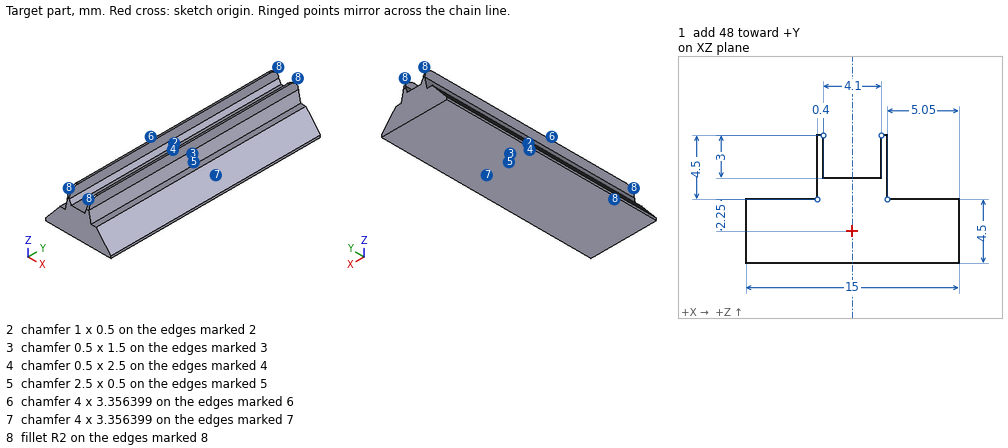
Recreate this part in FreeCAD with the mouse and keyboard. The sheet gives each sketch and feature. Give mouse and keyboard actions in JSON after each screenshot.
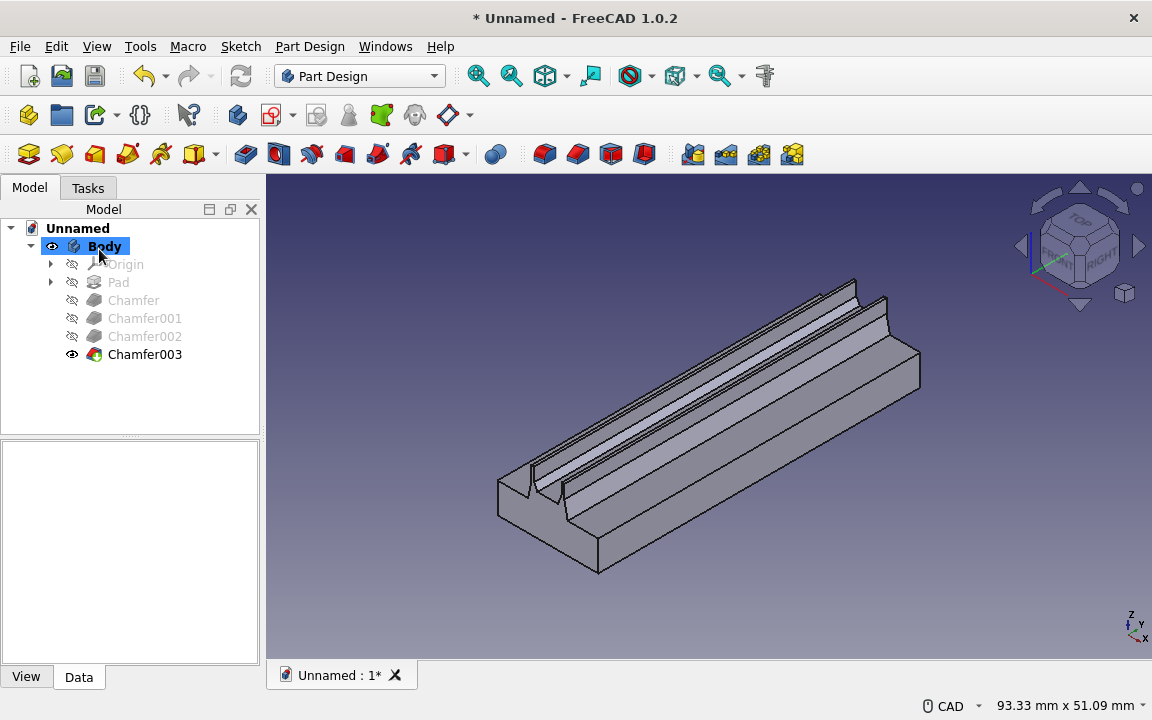
{"action": "key", "text": "2"}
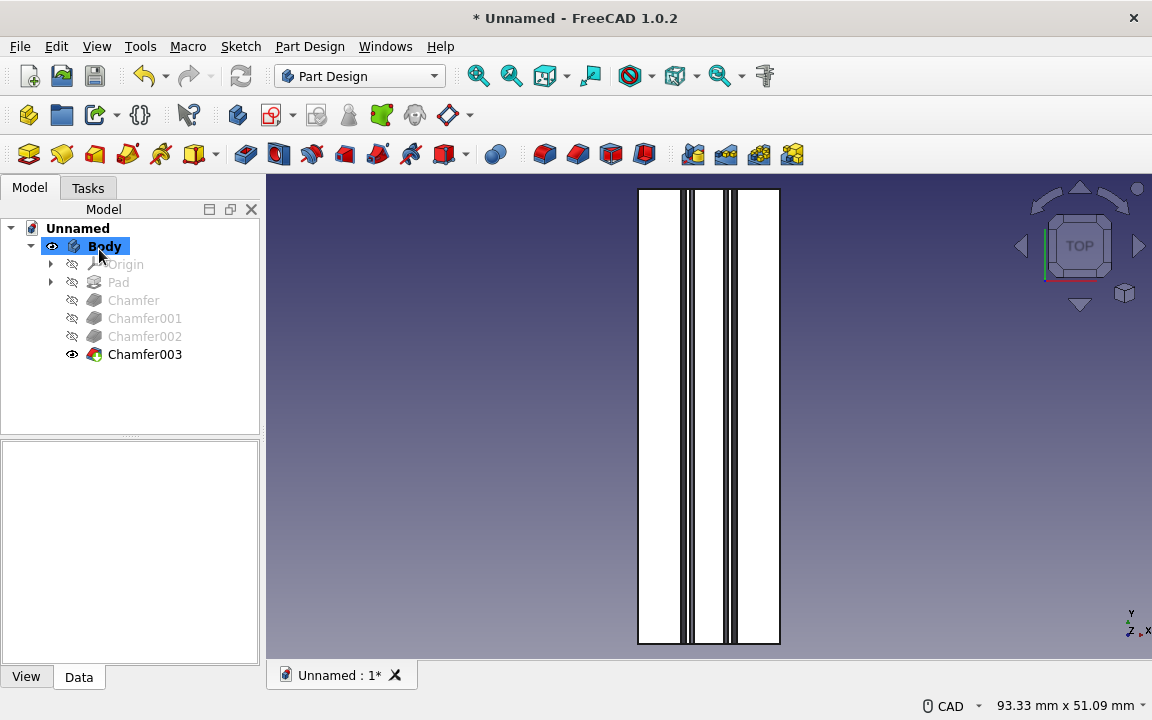
{"action": "left_click", "coordinate": [638, 416]}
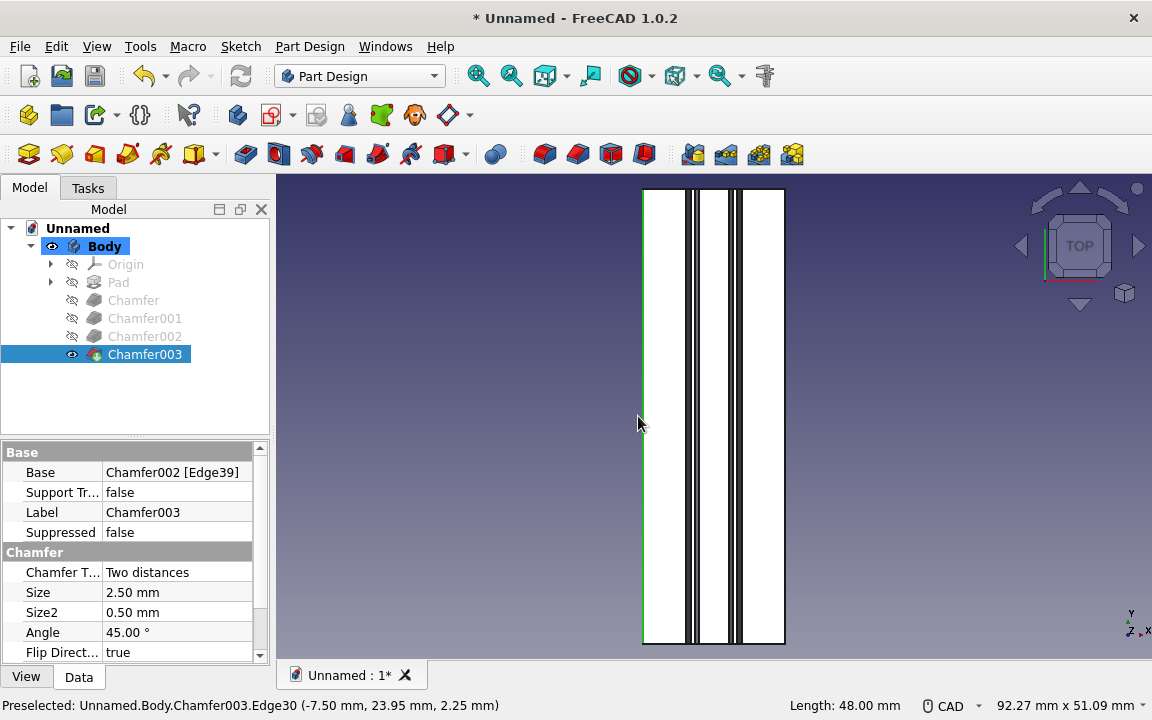
{"action": "left_click", "coordinate": [578, 154]}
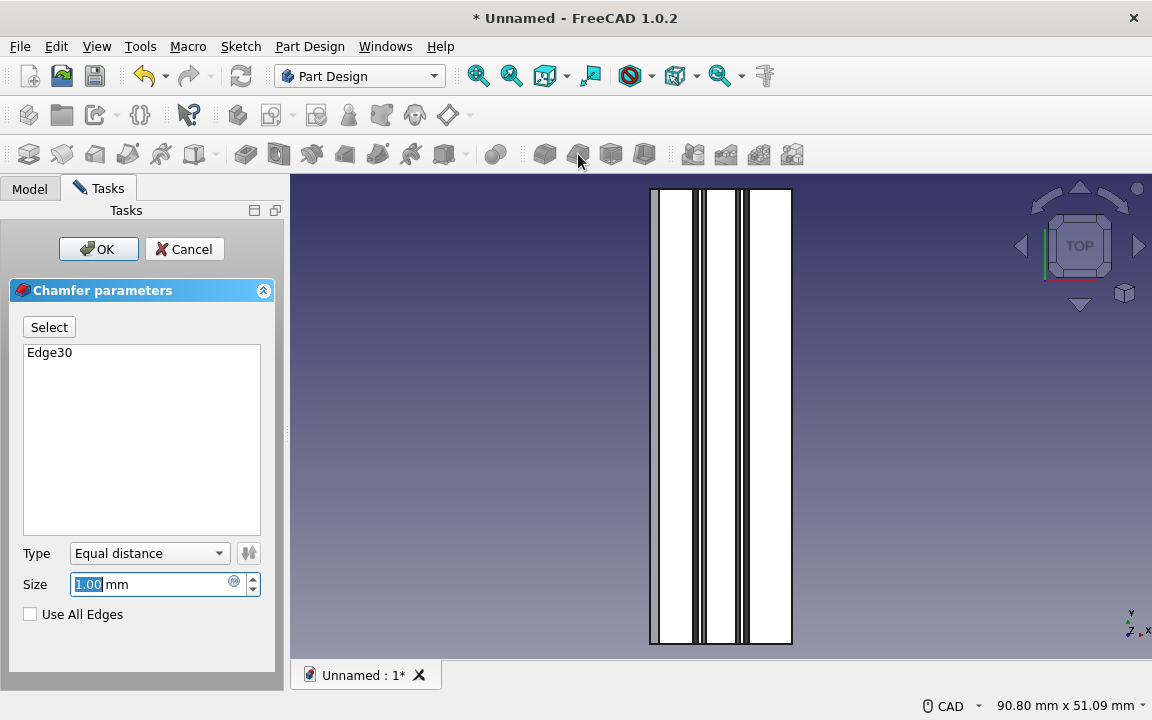
{"action": "type", "text": "4"}
{"action": "key", "text": "Tab"}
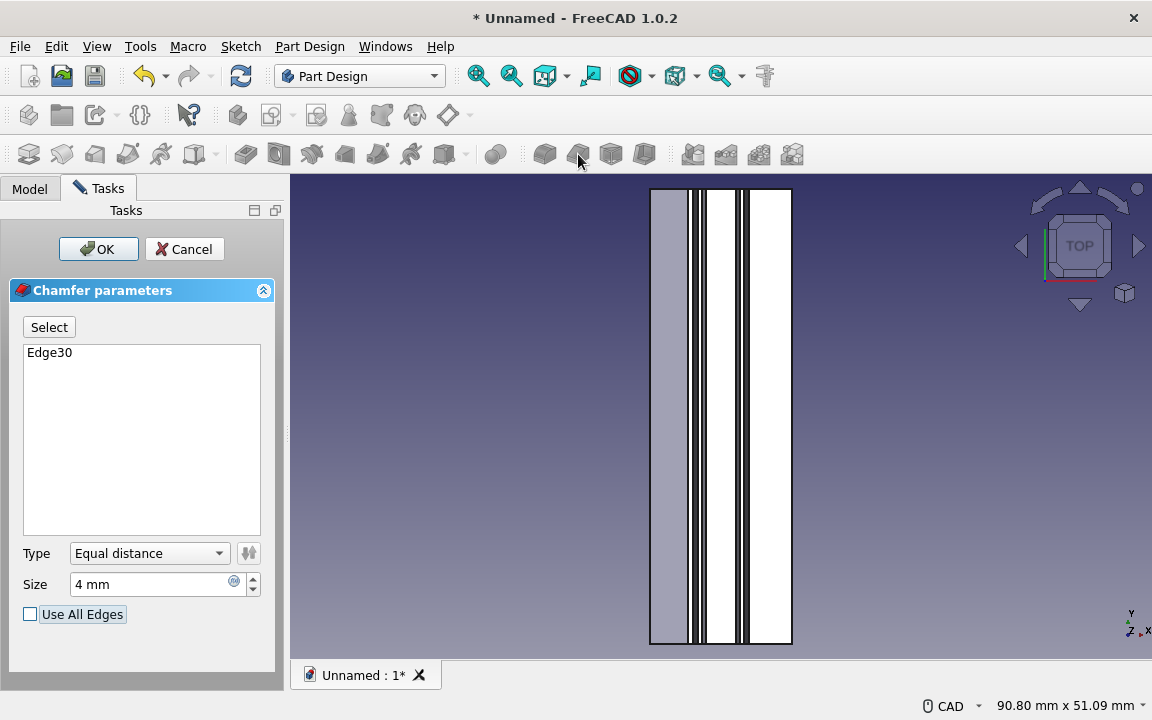
{"action": "left_click", "coordinate": [150, 554]}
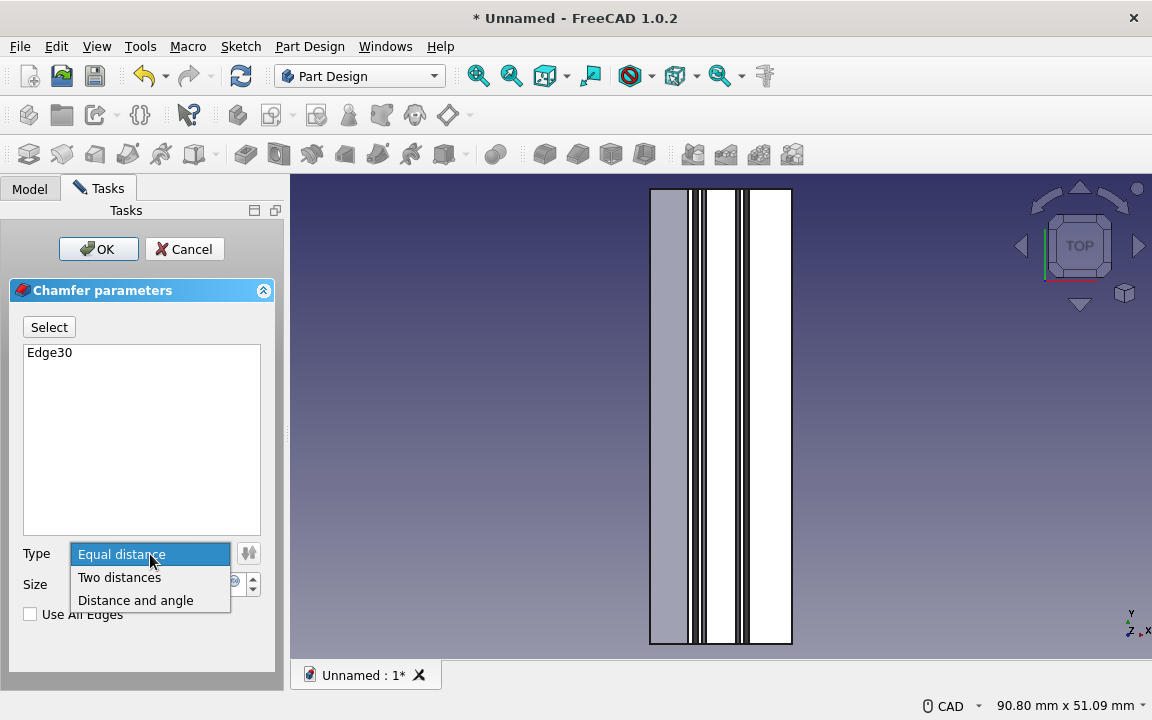
{"action": "left_click", "coordinate": [148, 578]}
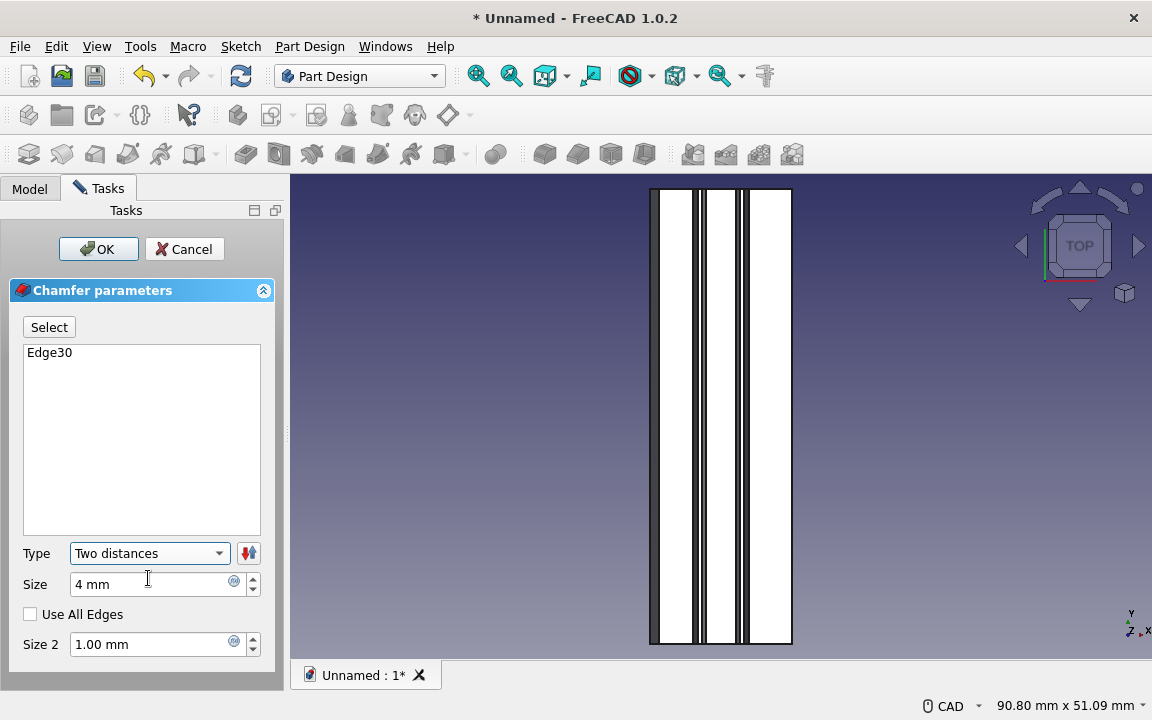
{"action": "triple_click", "coordinate": [158, 644]}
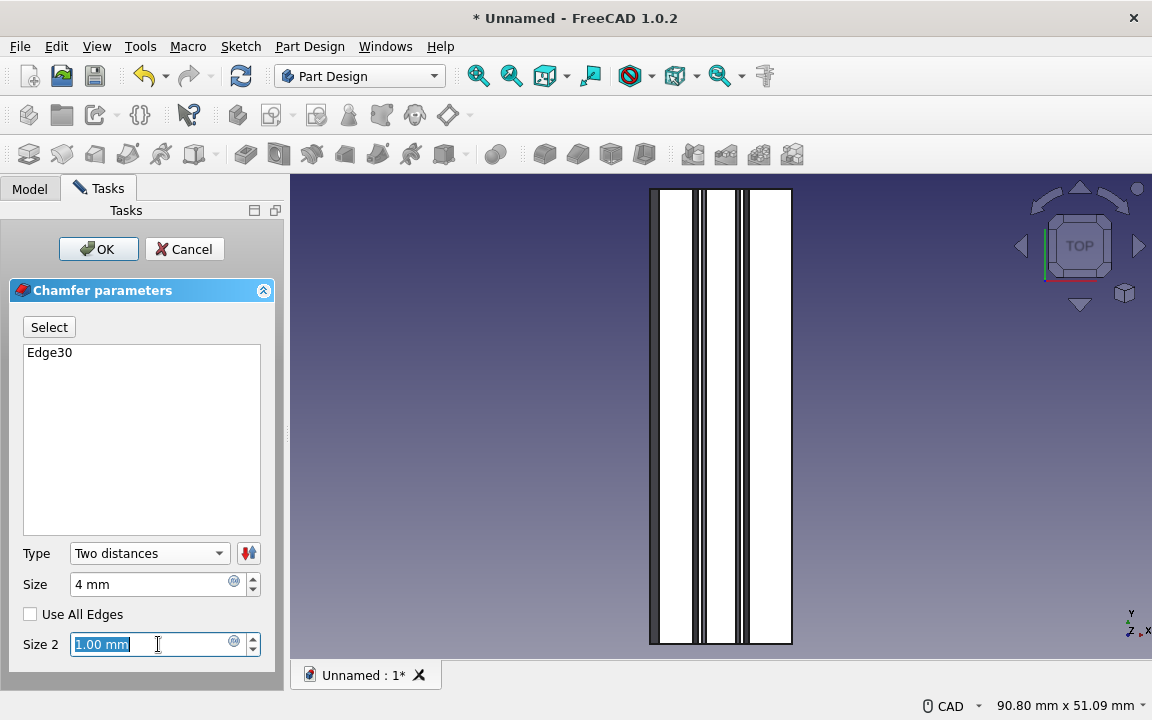
{"action": "type", "text": "3.356399"}
{"action": "key", "text": "Tab"}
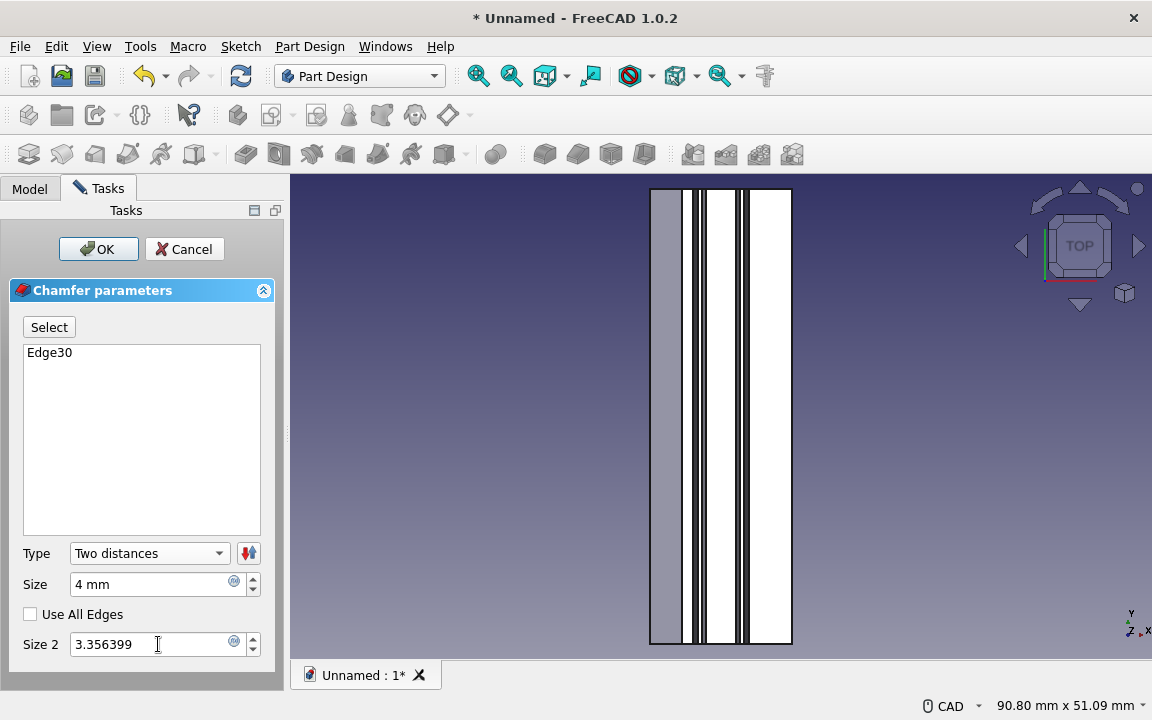
{"action": "left_click", "coordinate": [99, 249]}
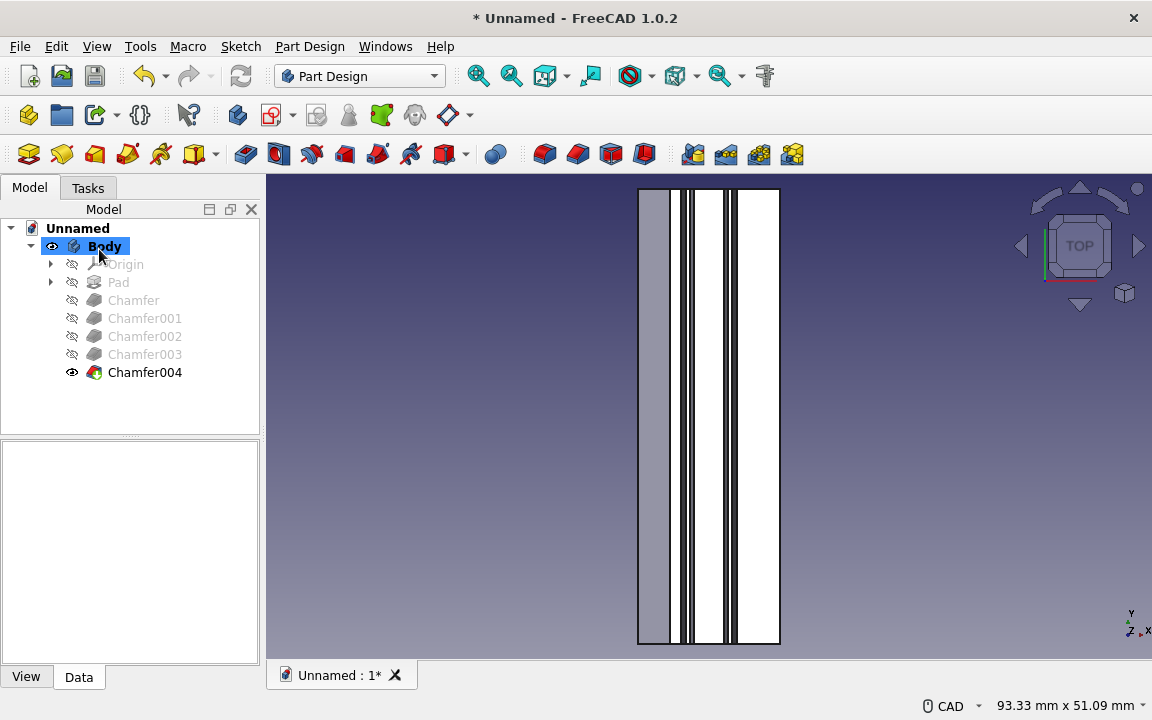
{"action": "left_click", "coordinate": [780, 416]}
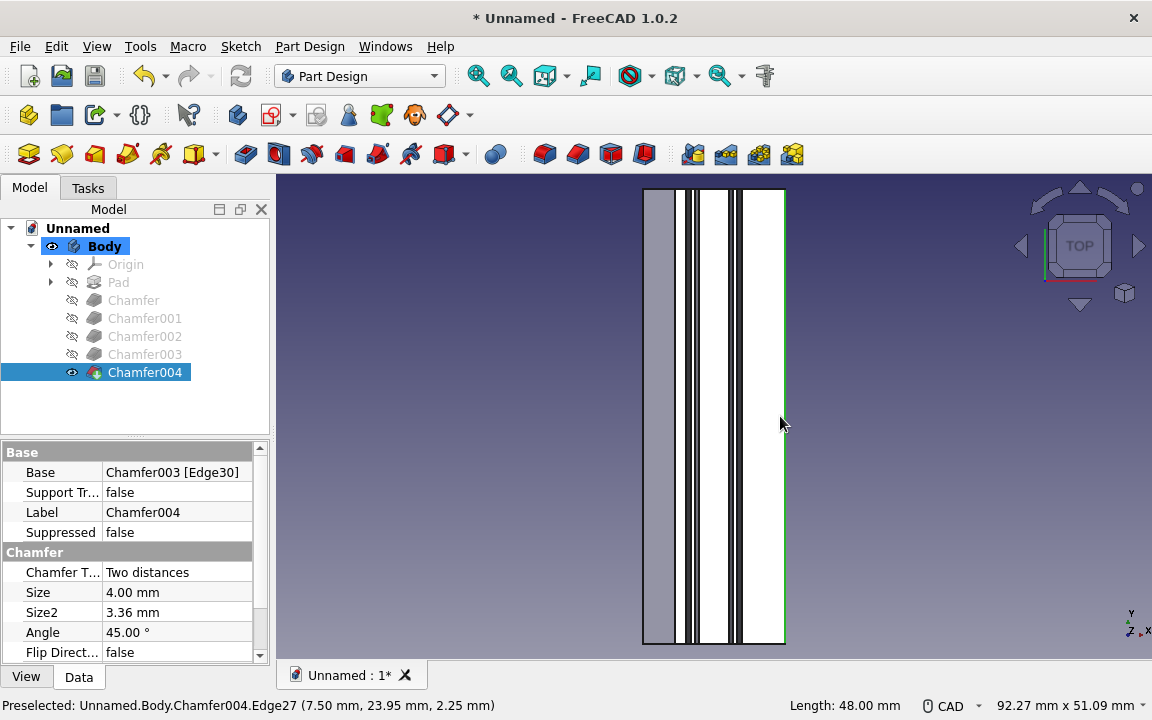
{"action": "left_click", "coordinate": [578, 154]}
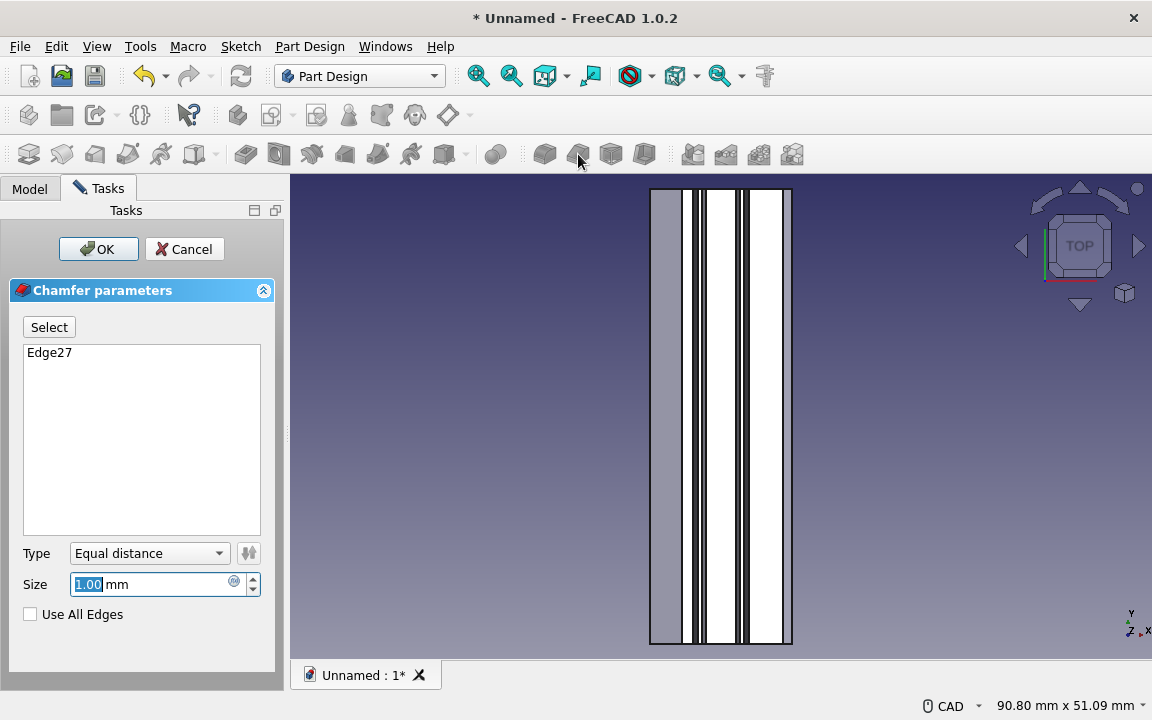
{"action": "type", "text": "4"}
{"action": "key", "text": "Tab"}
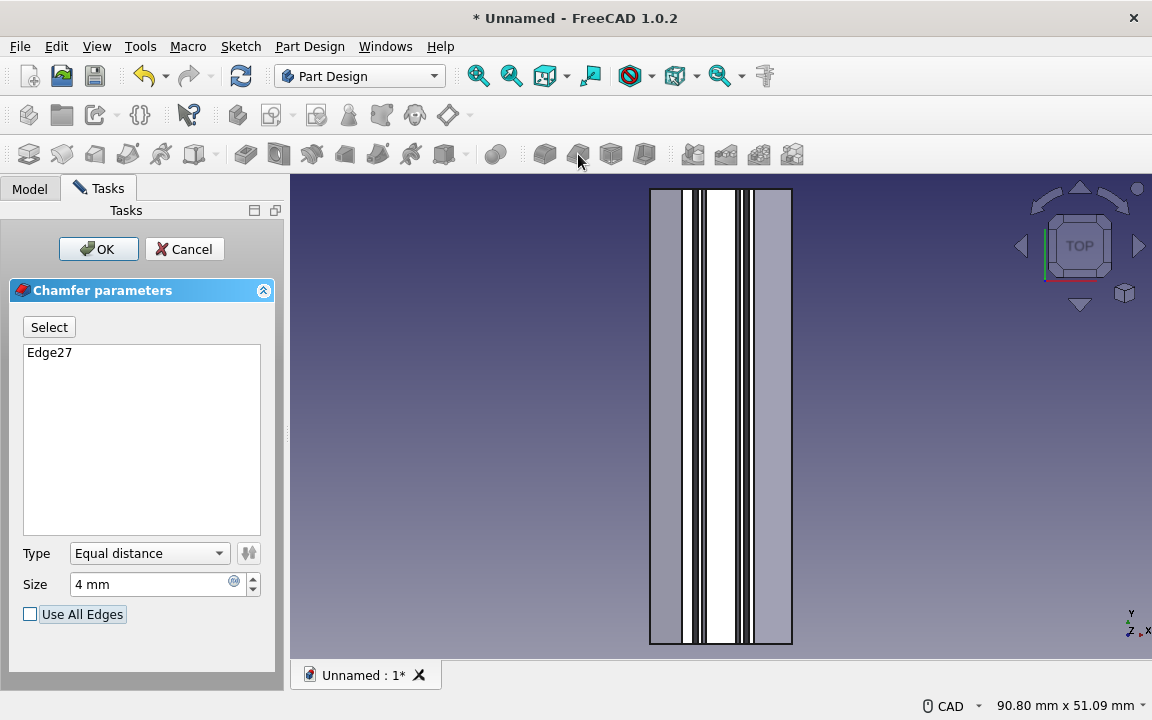
{"action": "left_click", "coordinate": [150, 554]}